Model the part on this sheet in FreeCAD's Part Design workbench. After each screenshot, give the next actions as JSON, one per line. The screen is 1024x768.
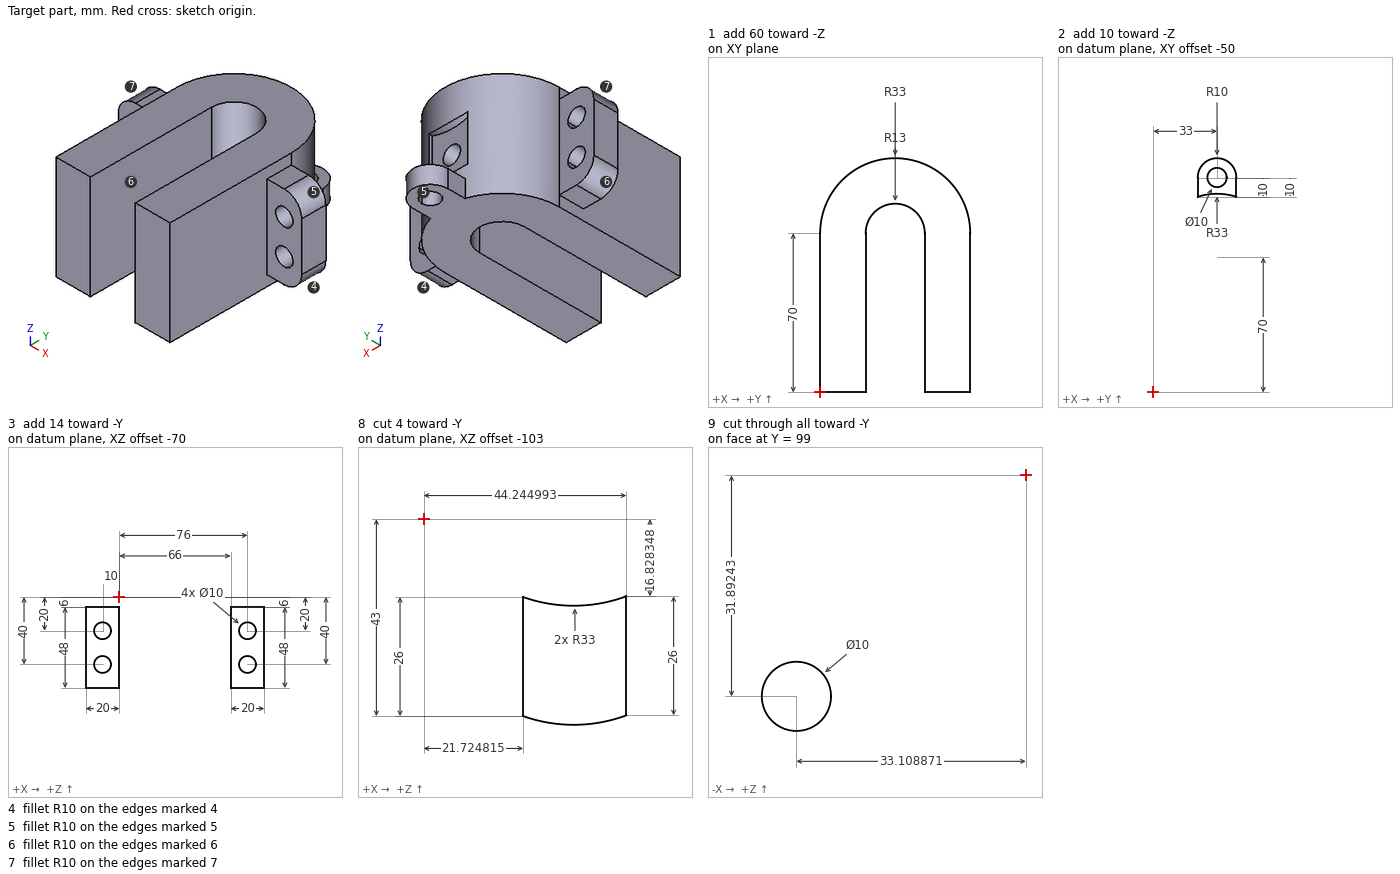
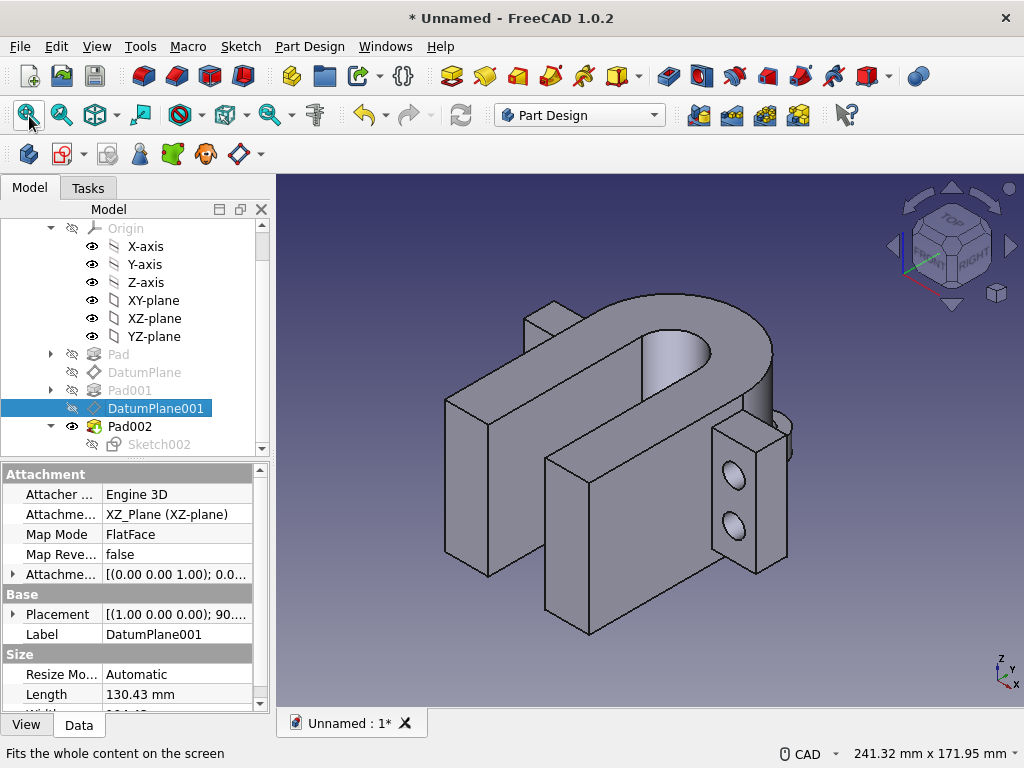
{"action": "key", "text": "2"}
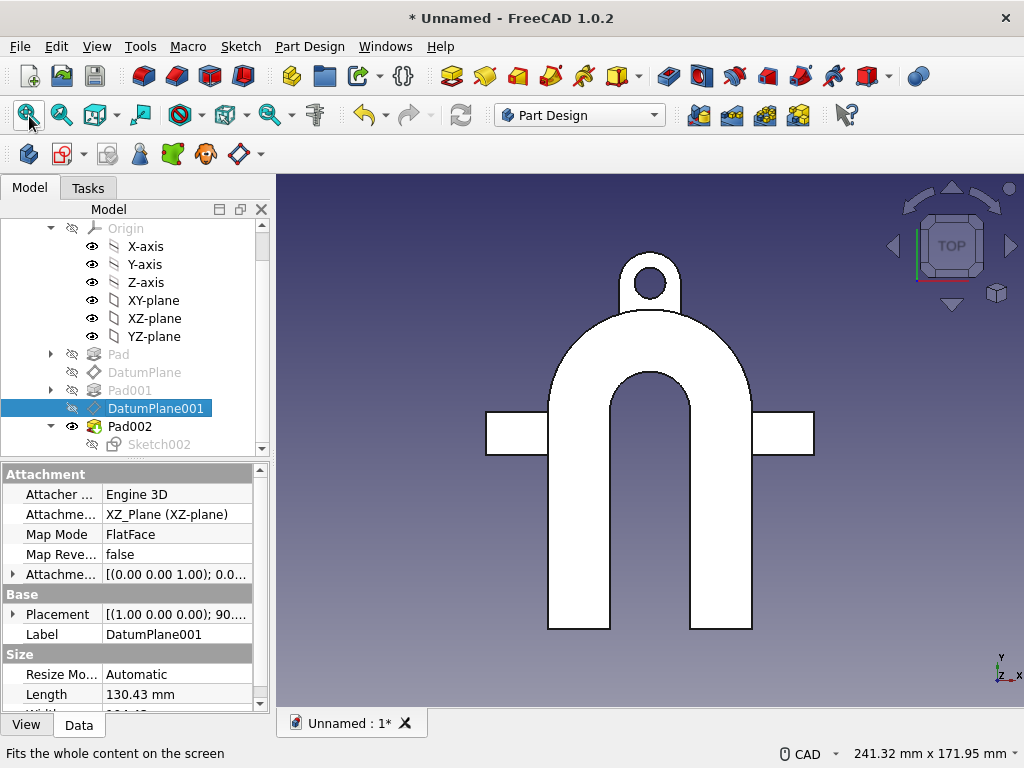
{"action": "key", "text": "1"}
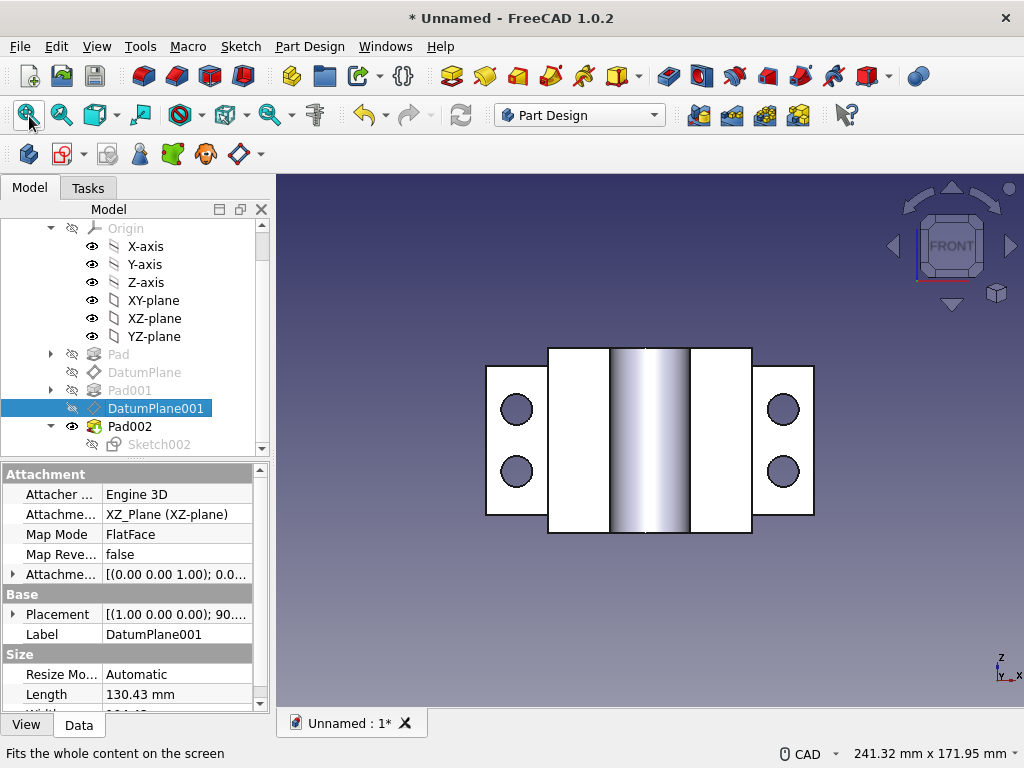
{"action": "key", "text": "v f"}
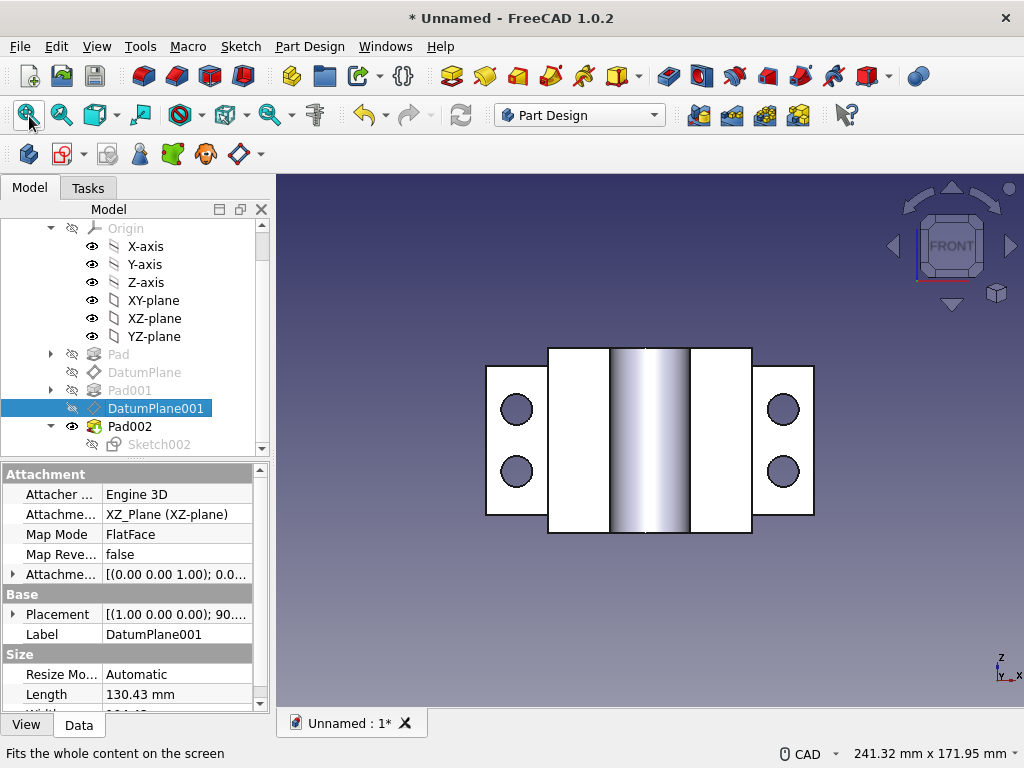
{"action": "key", "text": "3"}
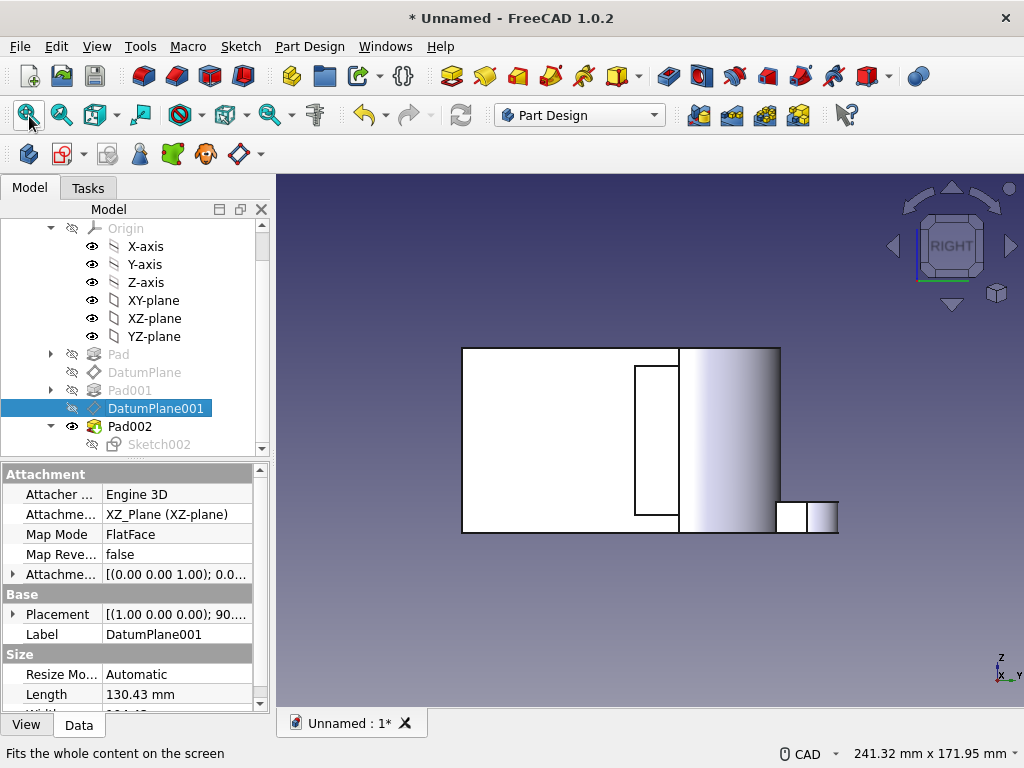
{"action": "left_click", "coordinate": [657, 514]}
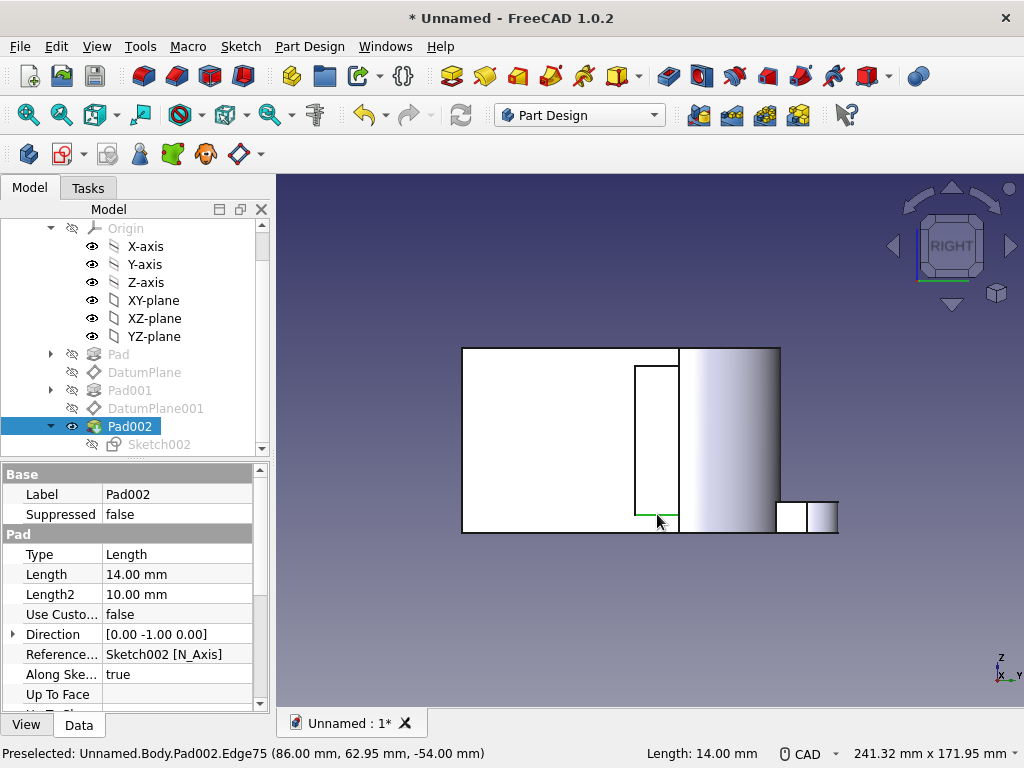
{"action": "left_click", "coordinate": [144, 76]}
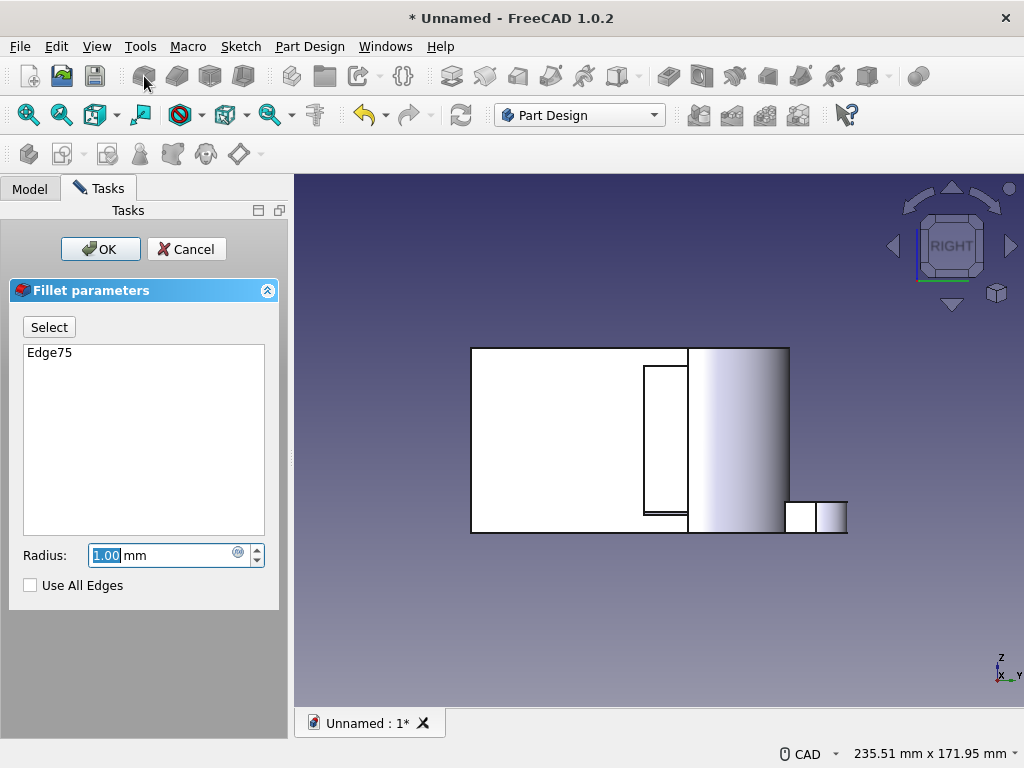
{"action": "type", "text": "10"}
{"action": "key", "text": "Tab"}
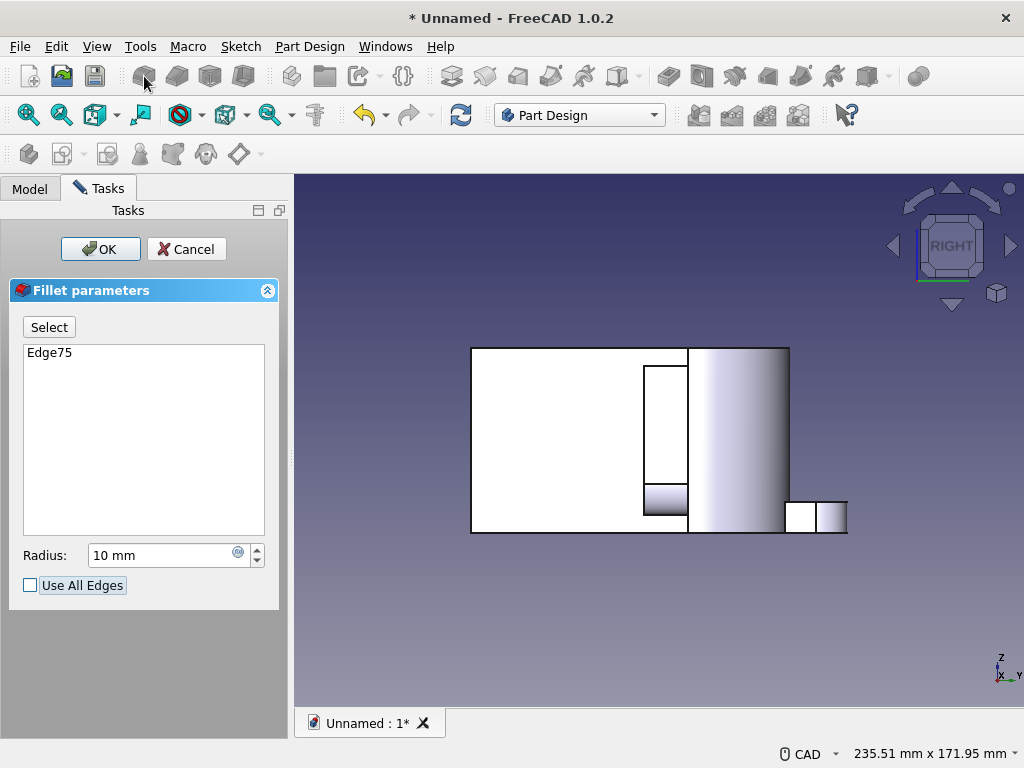
{"action": "left_click", "coordinate": [101, 249]}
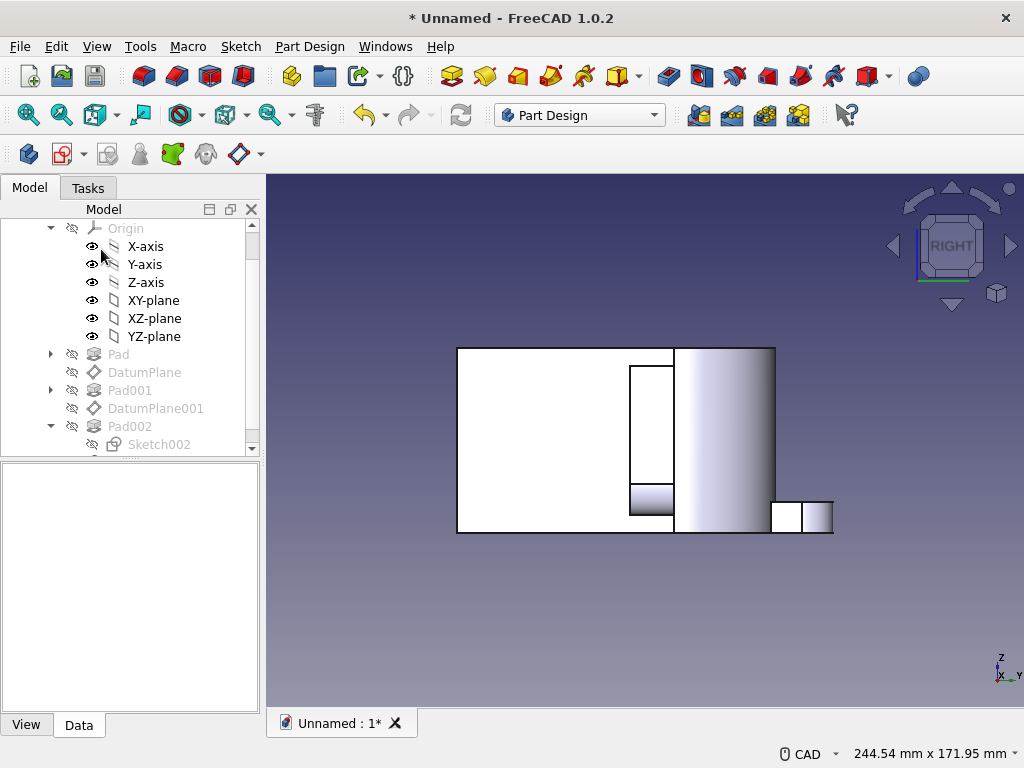
{"action": "left_click", "coordinate": [652, 365]}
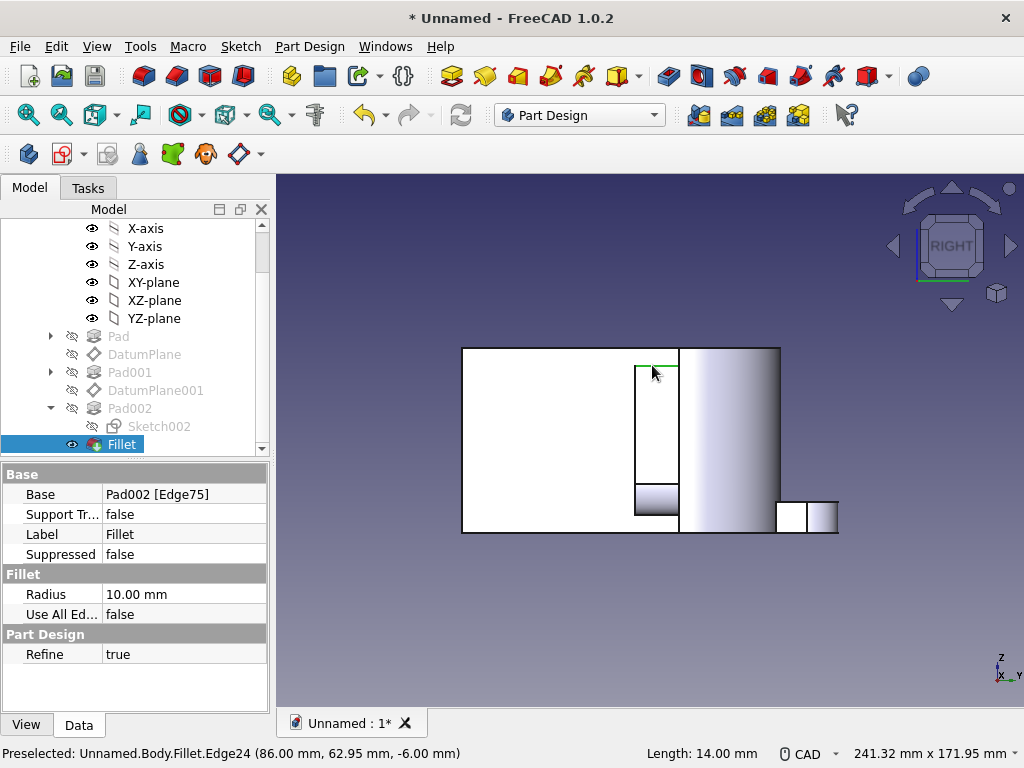
{"action": "left_click", "coordinate": [144, 76]}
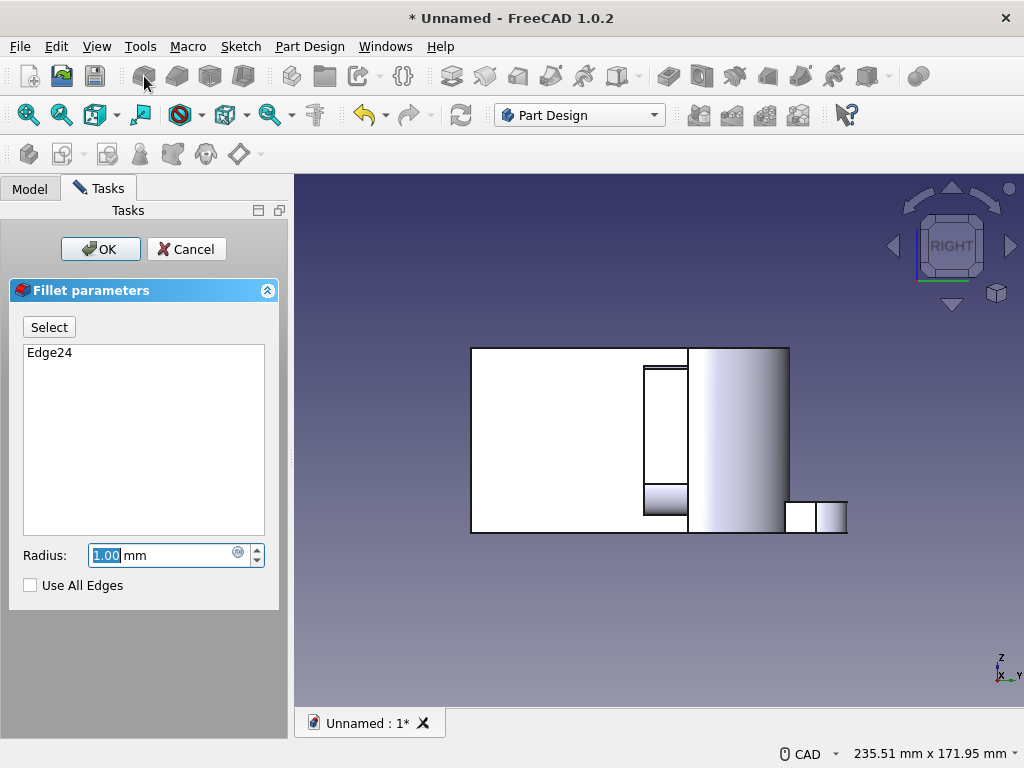
{"action": "type", "text": "10"}
{"action": "key", "text": "Tab"}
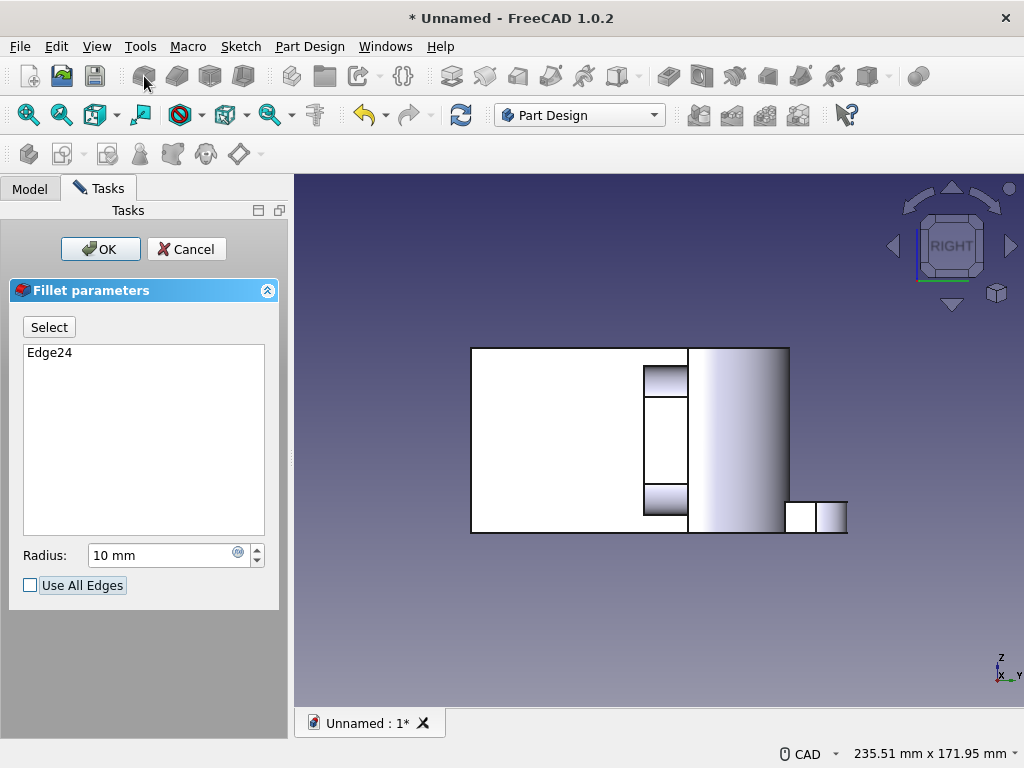
{"action": "left_click", "coordinate": [101, 249]}